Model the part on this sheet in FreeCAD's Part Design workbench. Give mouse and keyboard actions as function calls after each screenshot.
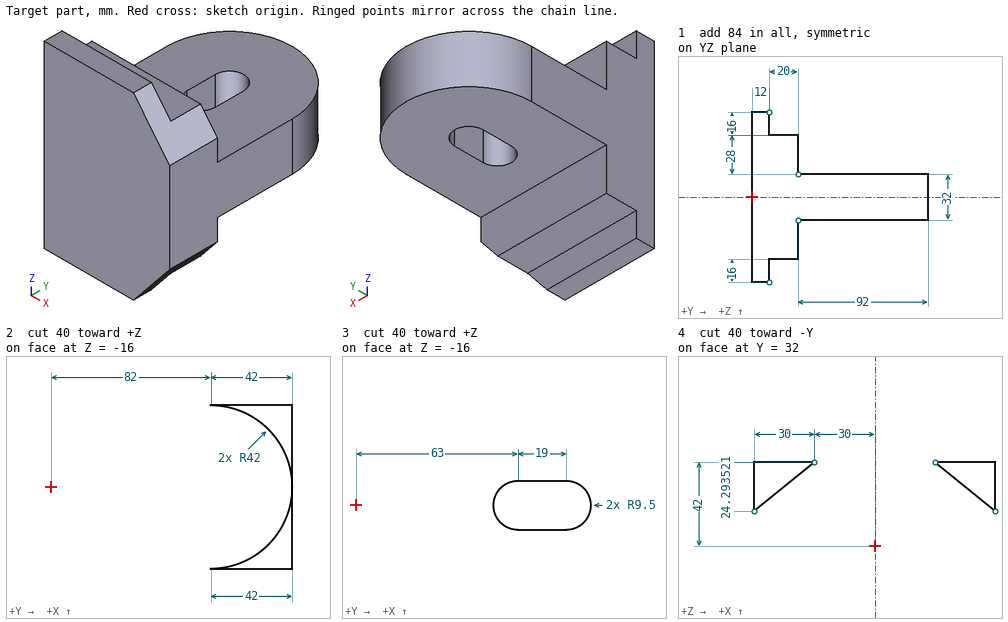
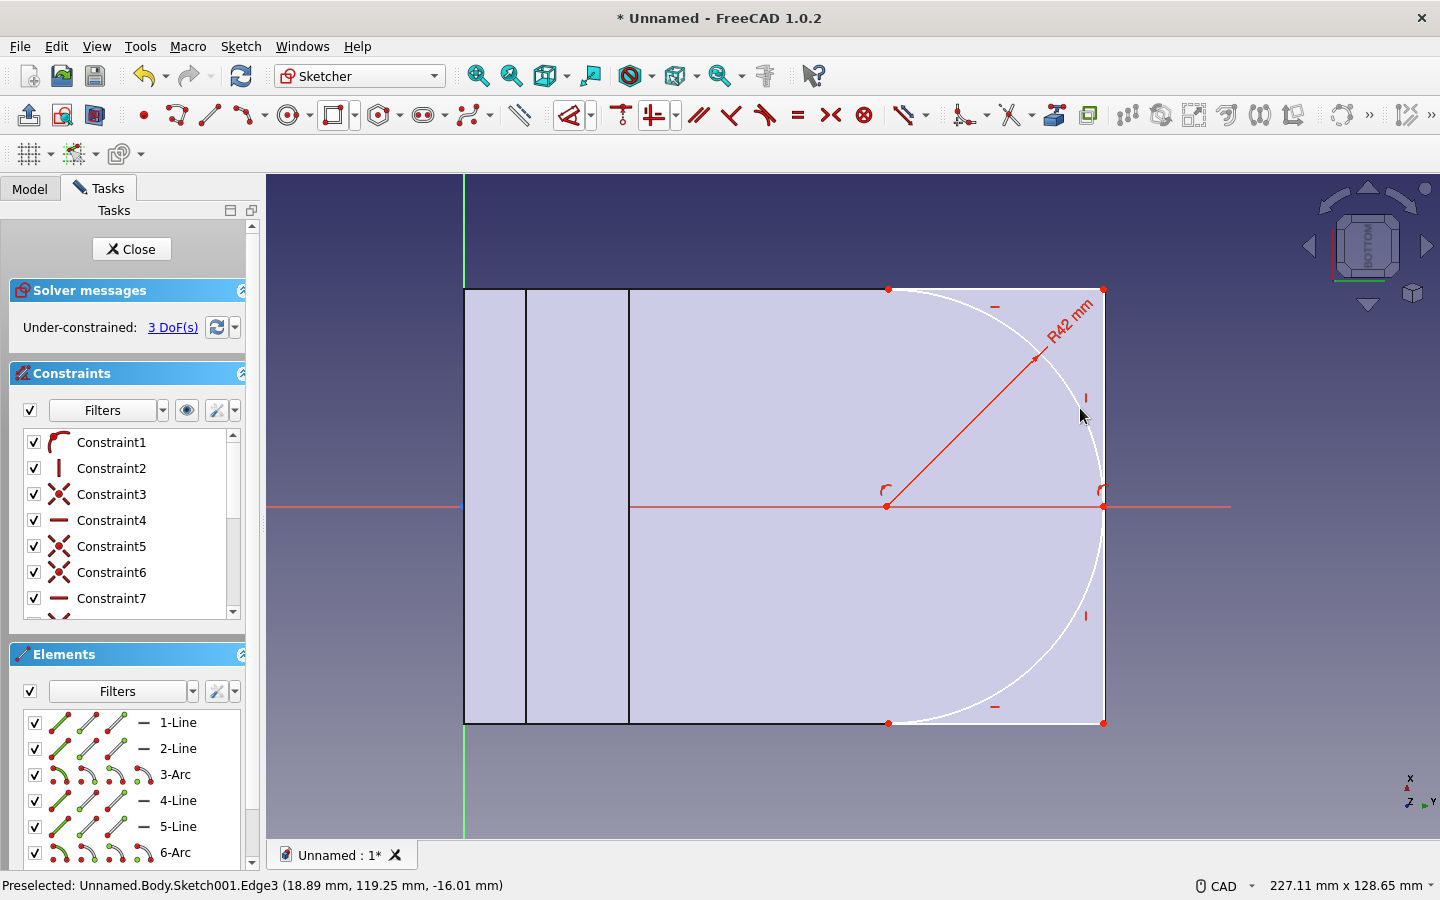
click(1039, 289)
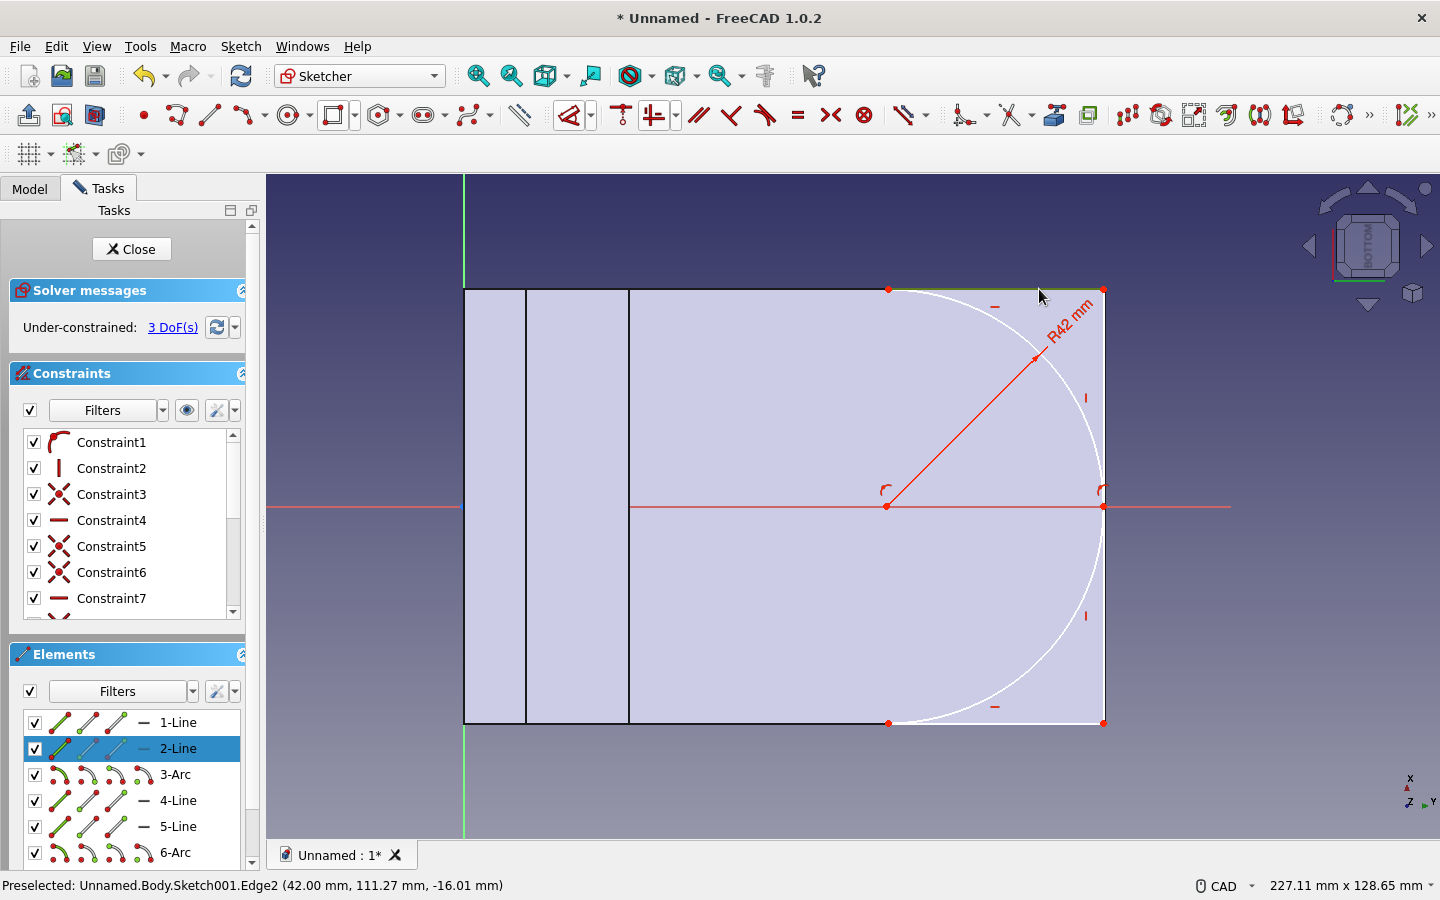
key(l)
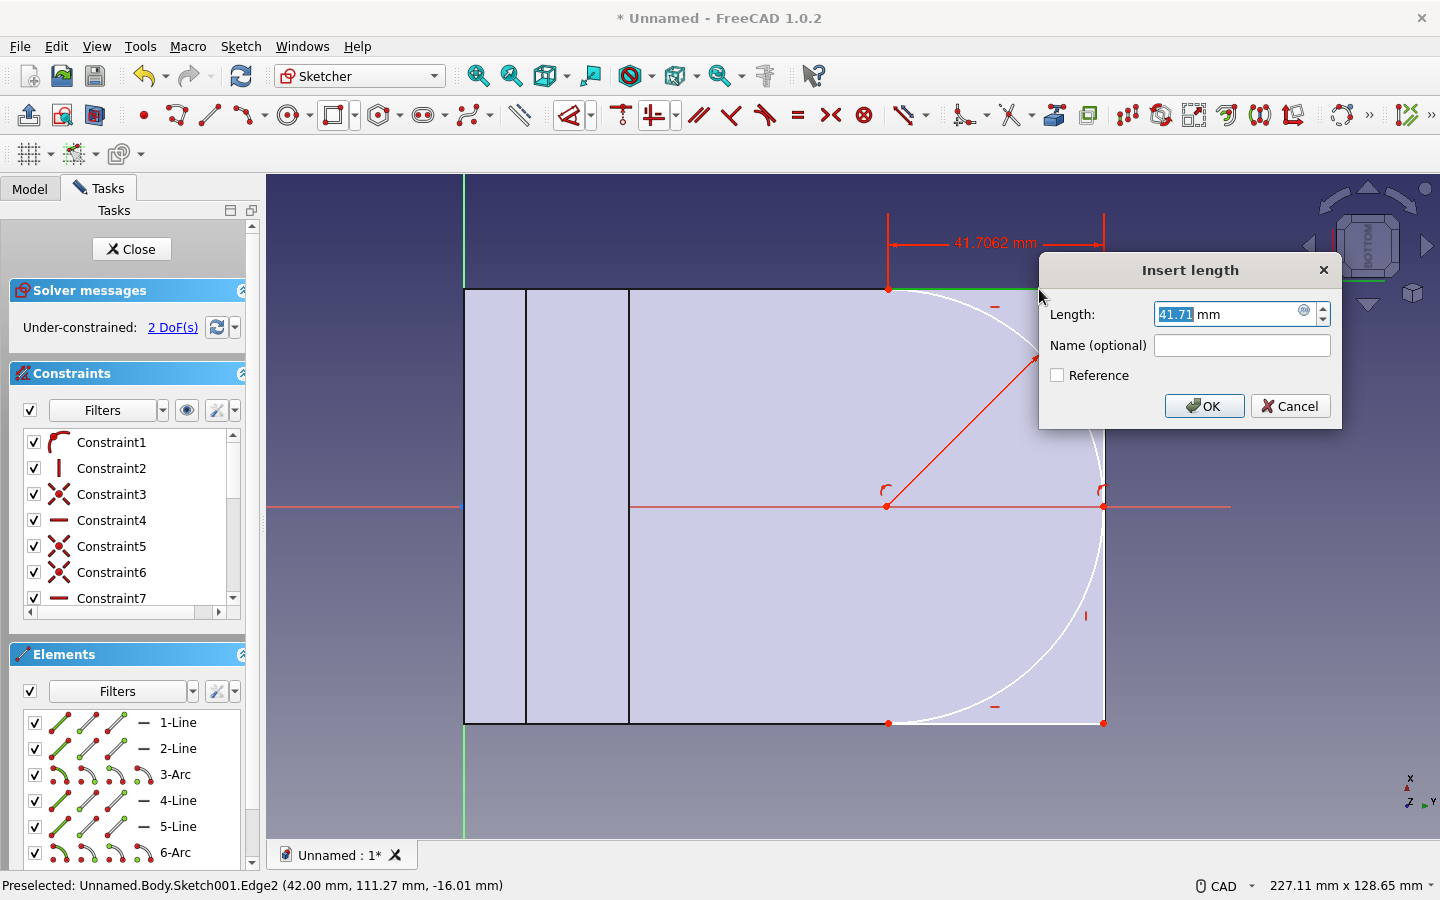
text(42)
key(Return)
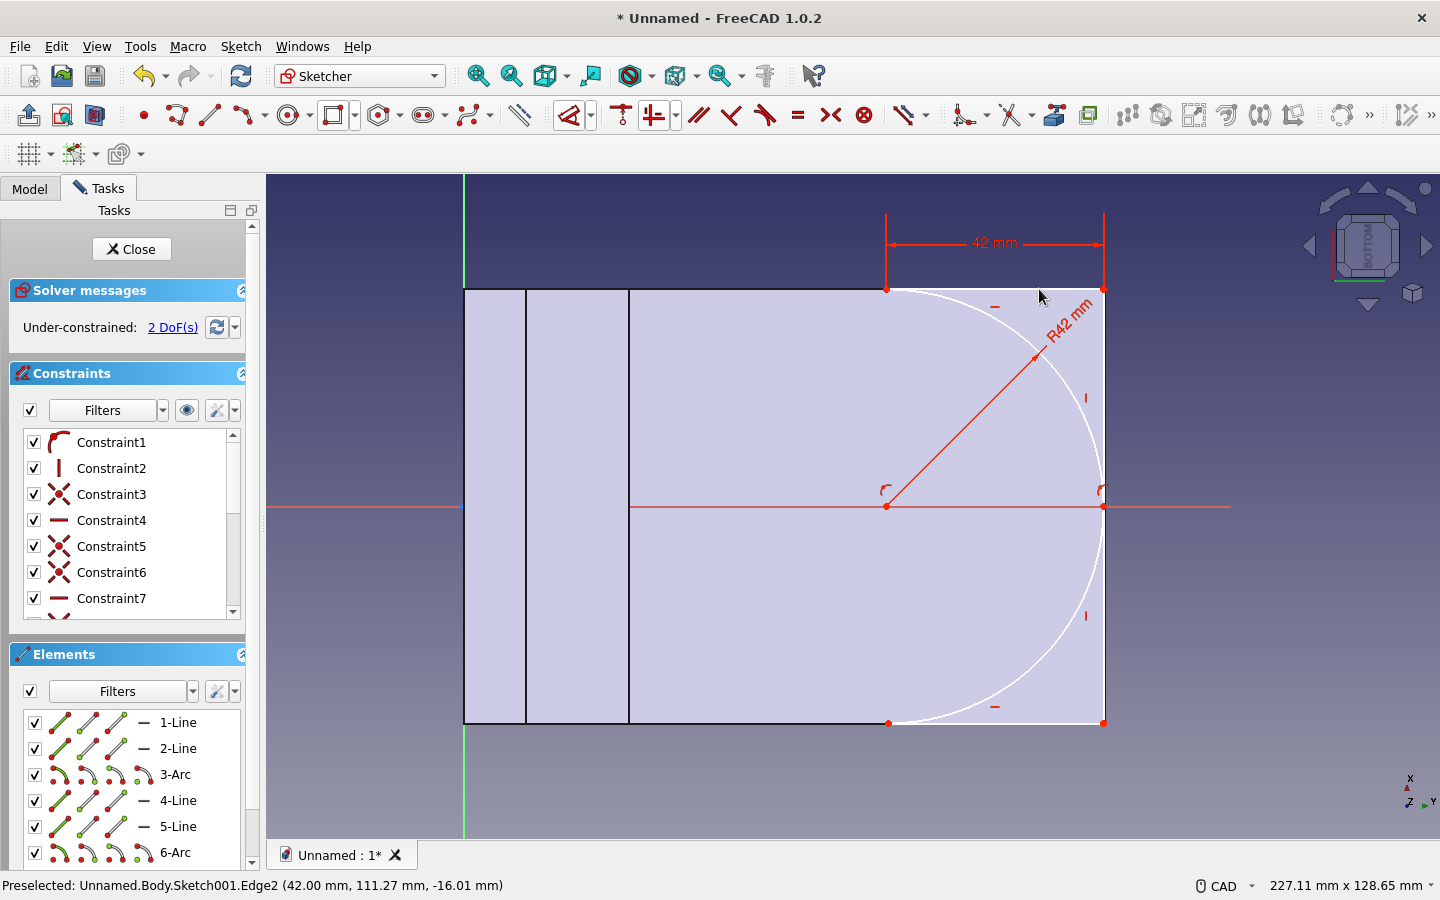
scroll(953, 724, up, 2)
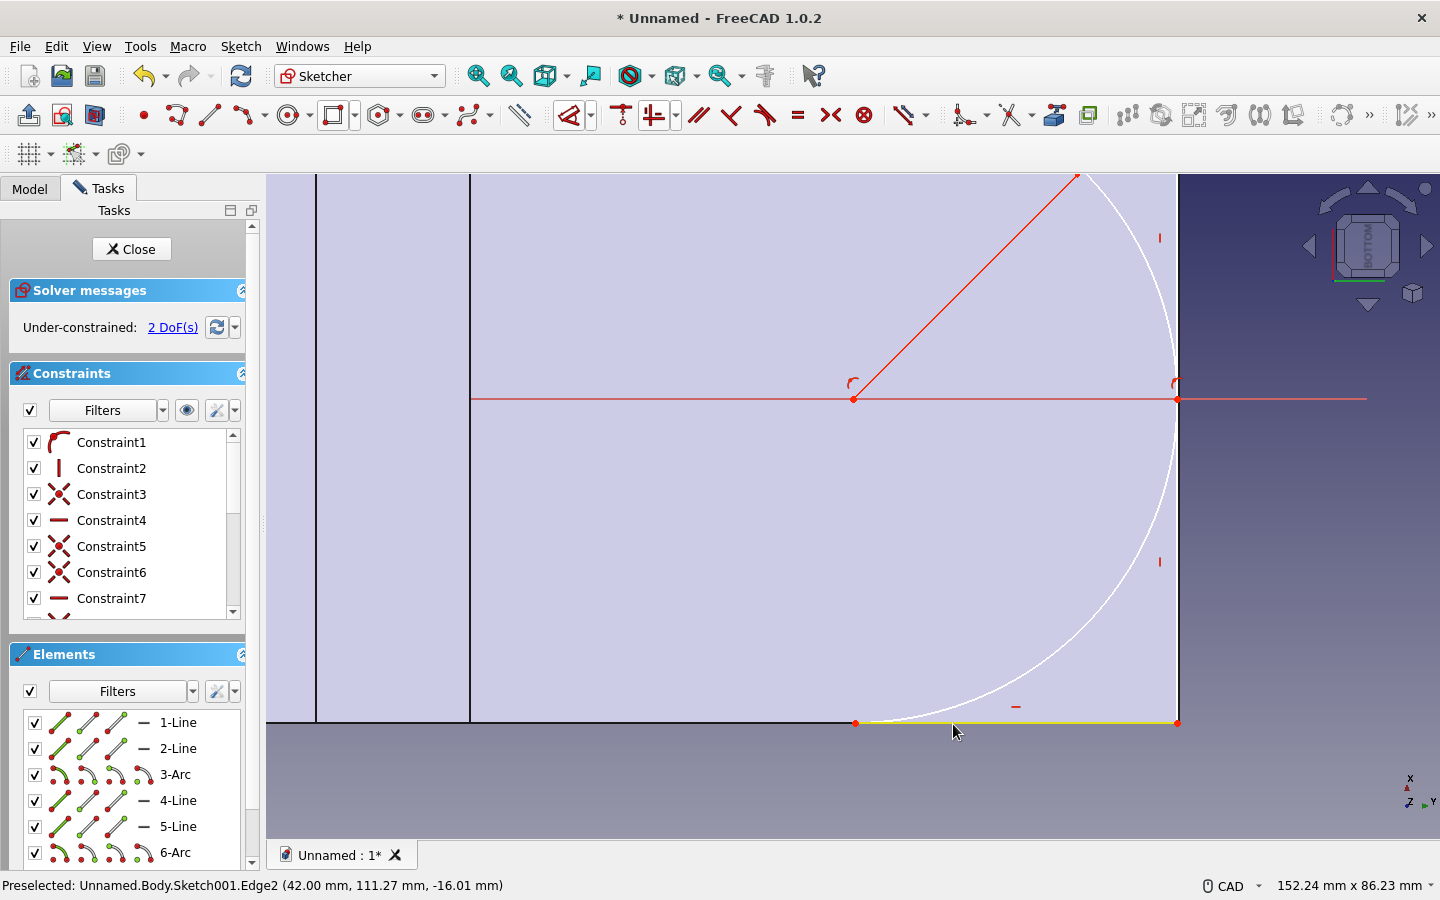
click(952, 723)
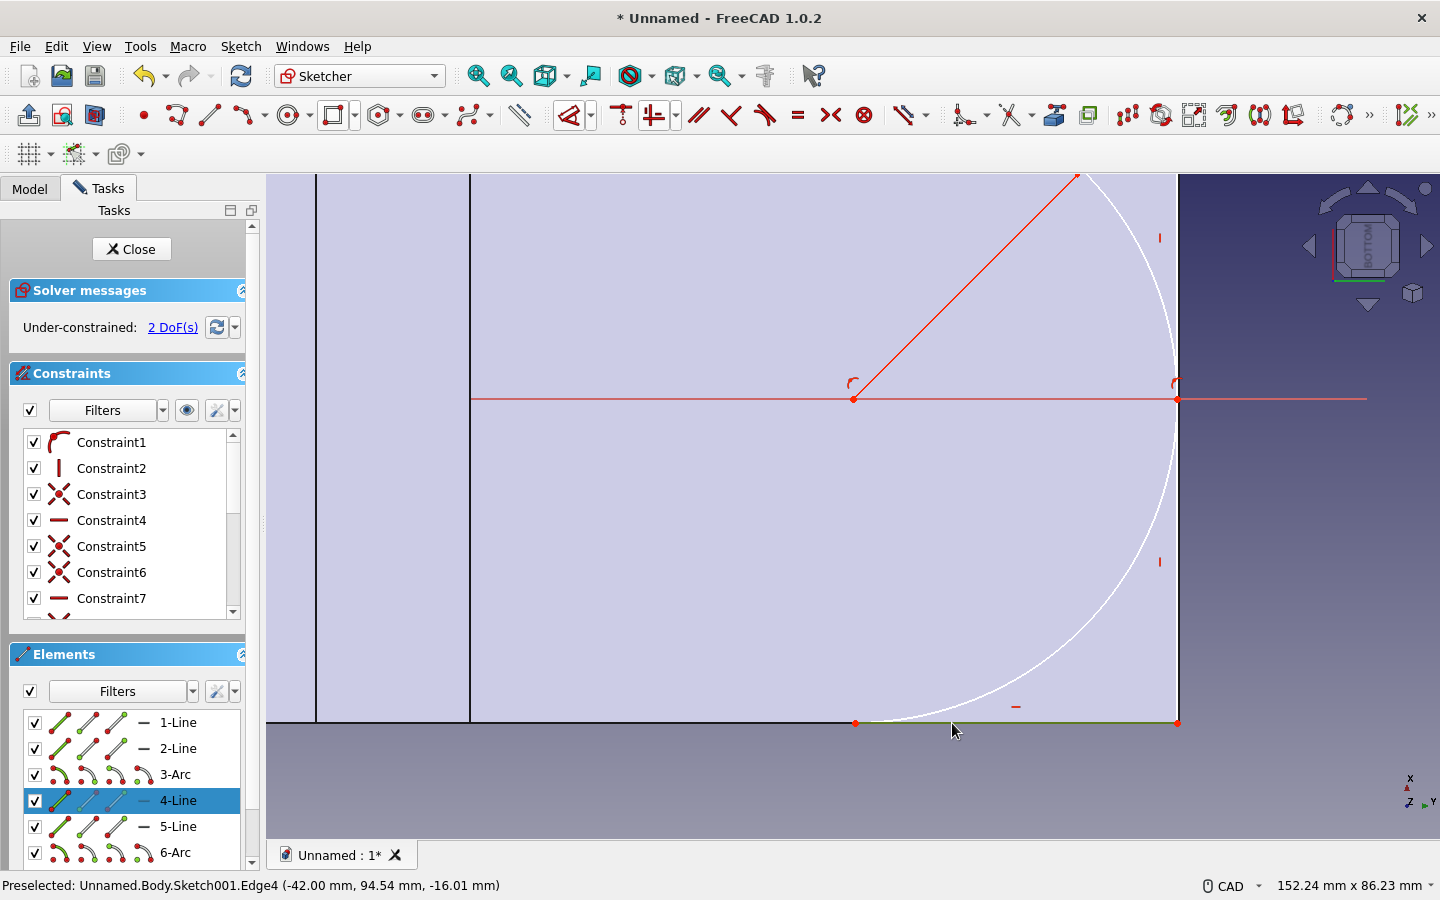
key(l)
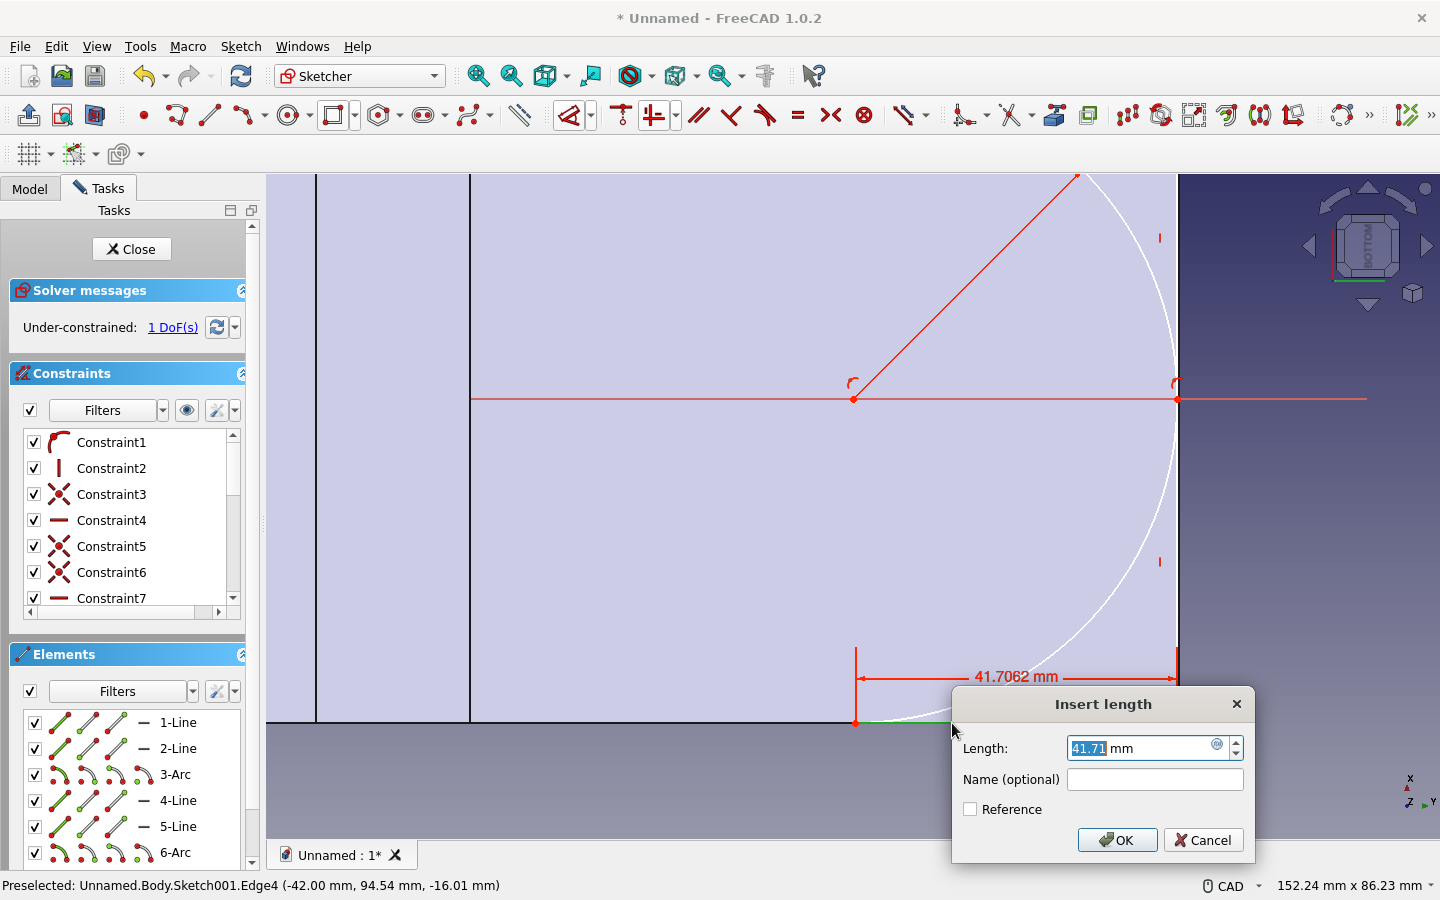
text(42)
key(Return)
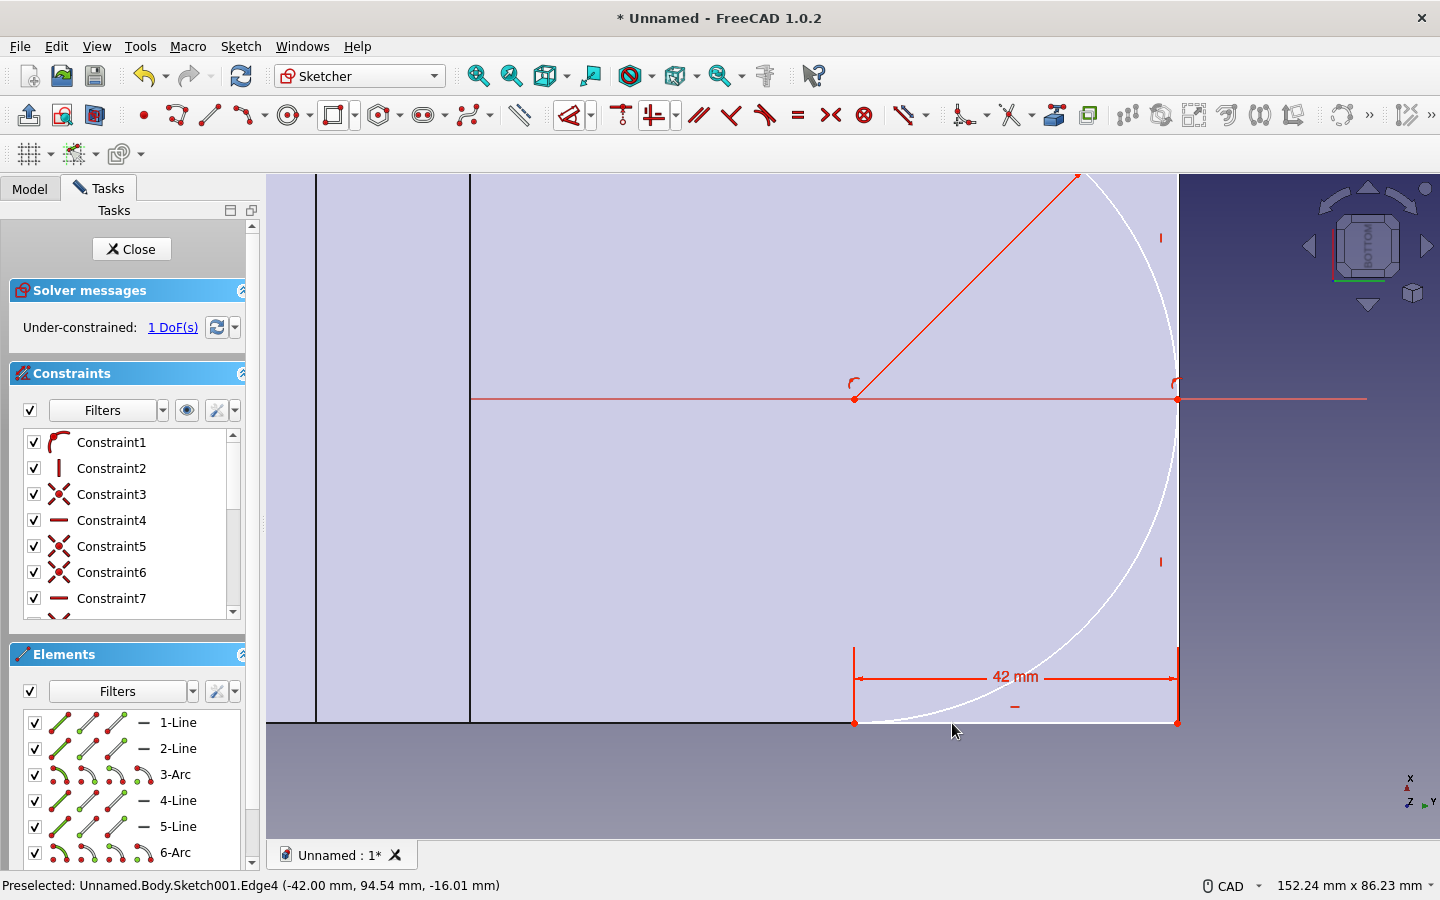
scroll(954, 725, down, 2)